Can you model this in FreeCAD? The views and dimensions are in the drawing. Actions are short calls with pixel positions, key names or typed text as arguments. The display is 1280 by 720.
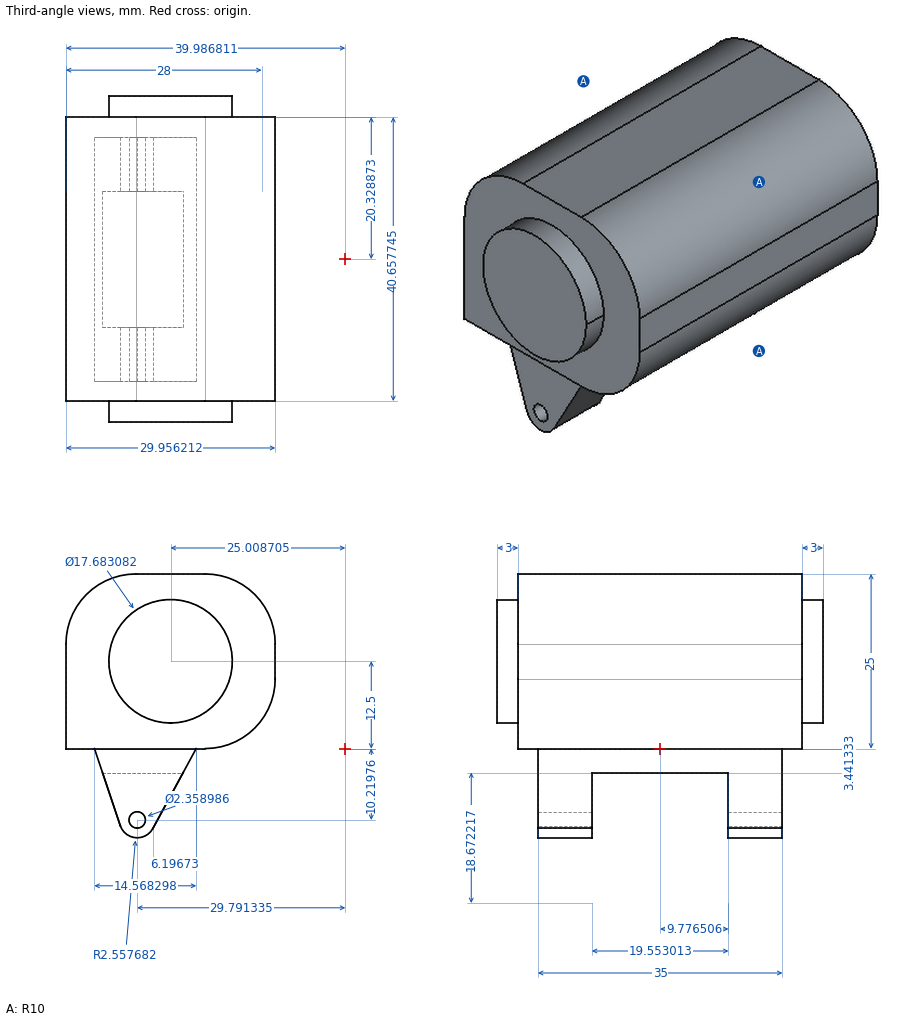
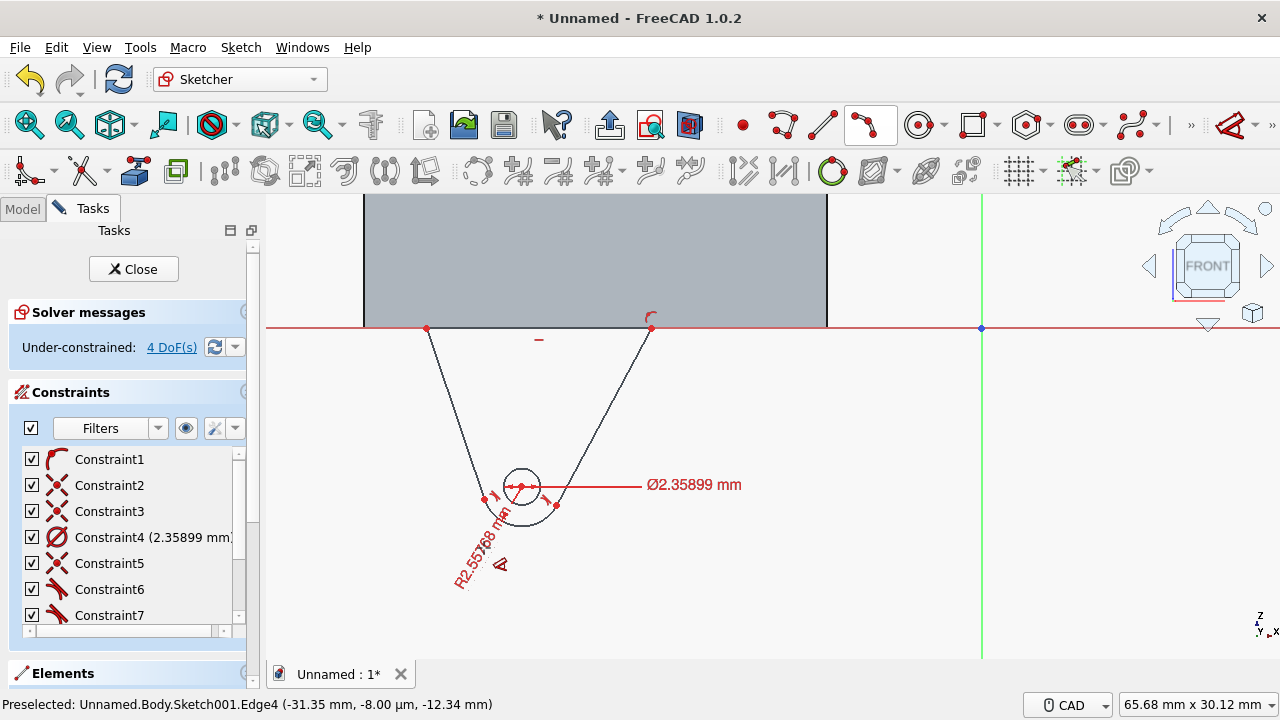
click(585, 452)
click(604, 294)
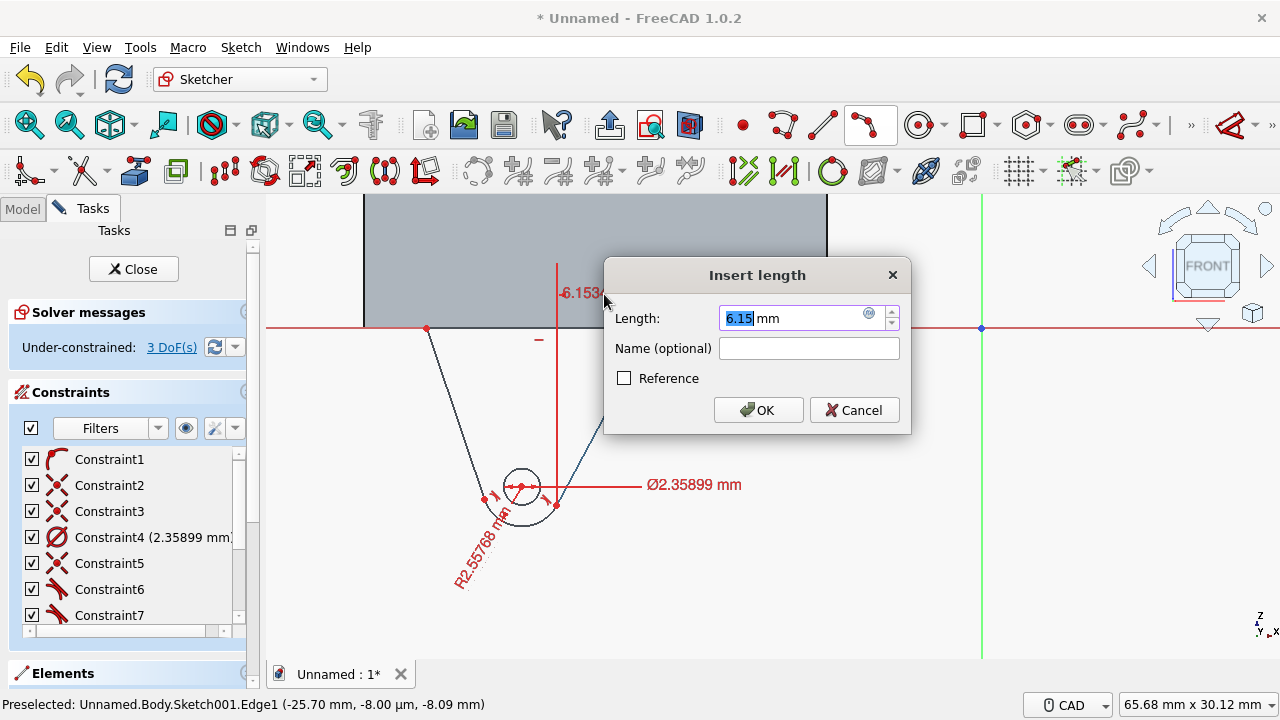
text(6.19673)
key(Return)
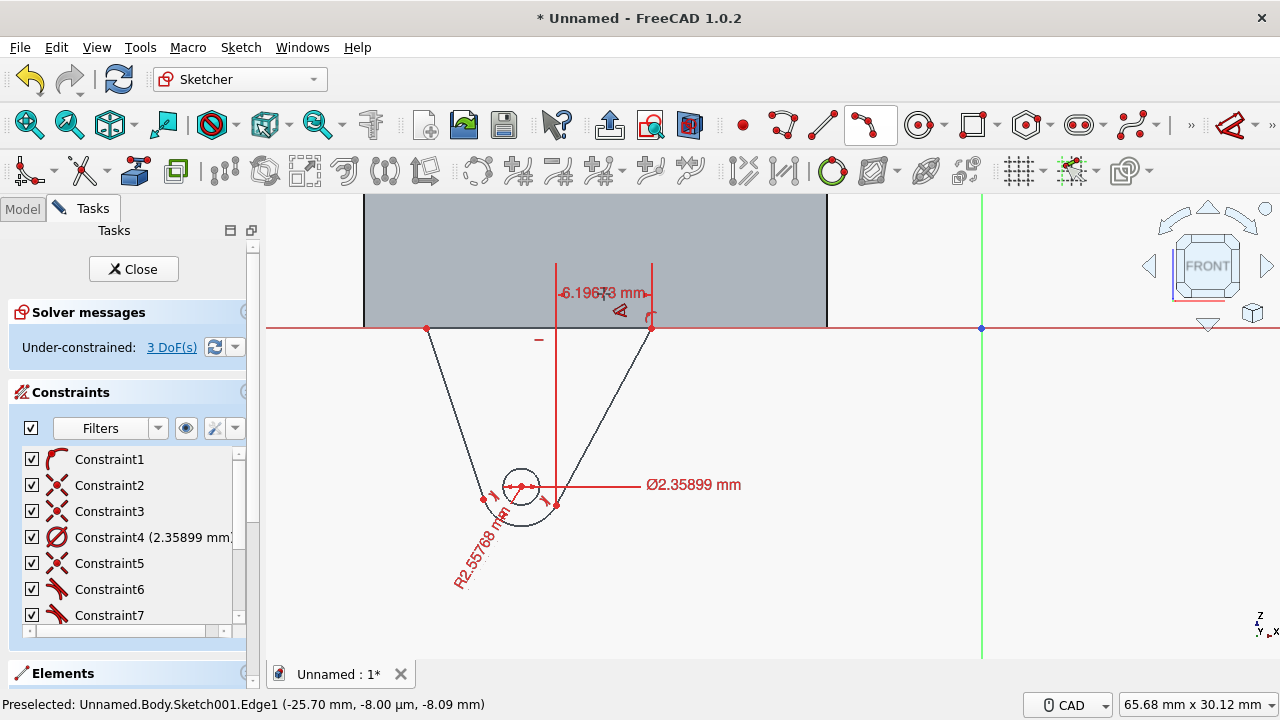
click(521, 487)
click(1016, 407)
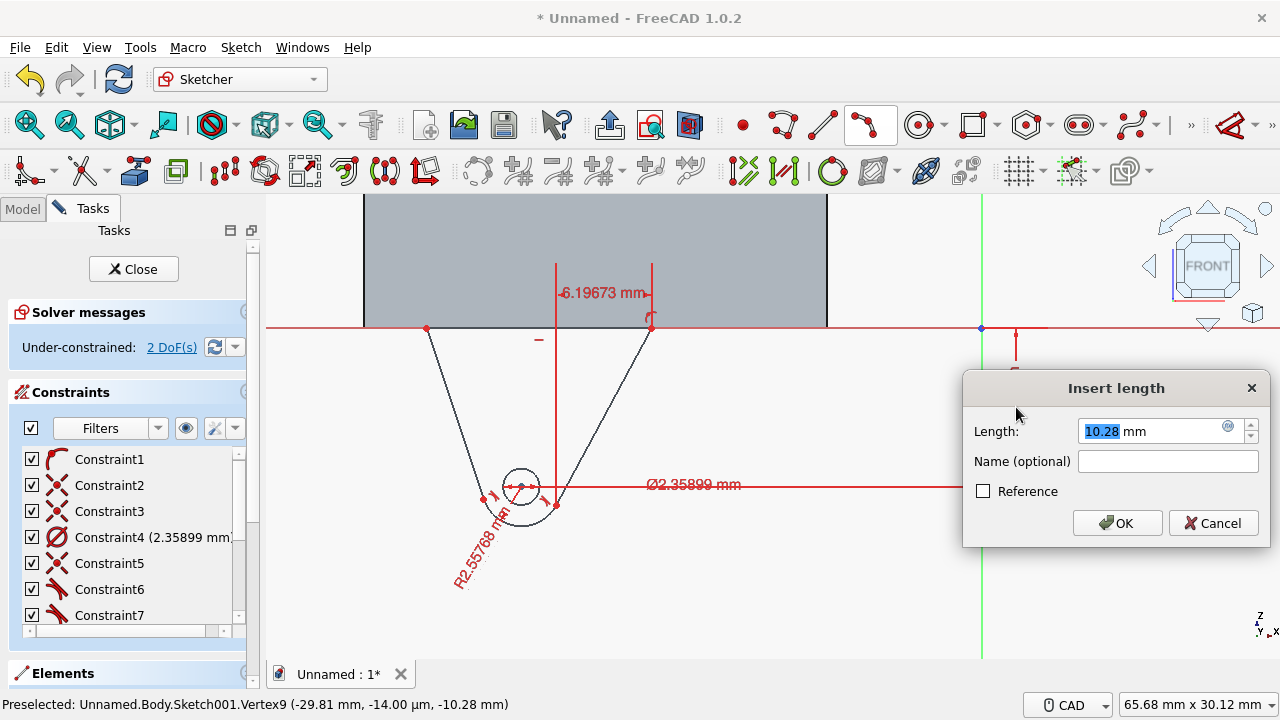
text(10.21976)
key(Return)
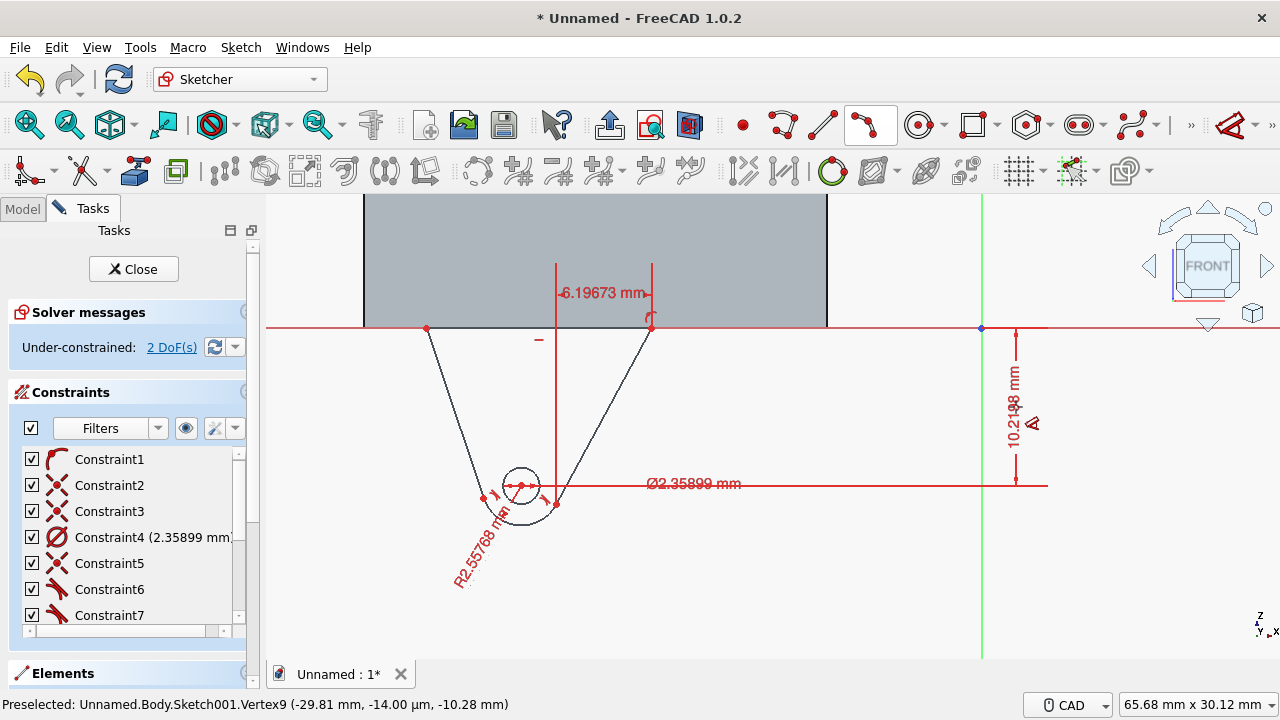
click(584, 328)
click(488, 294)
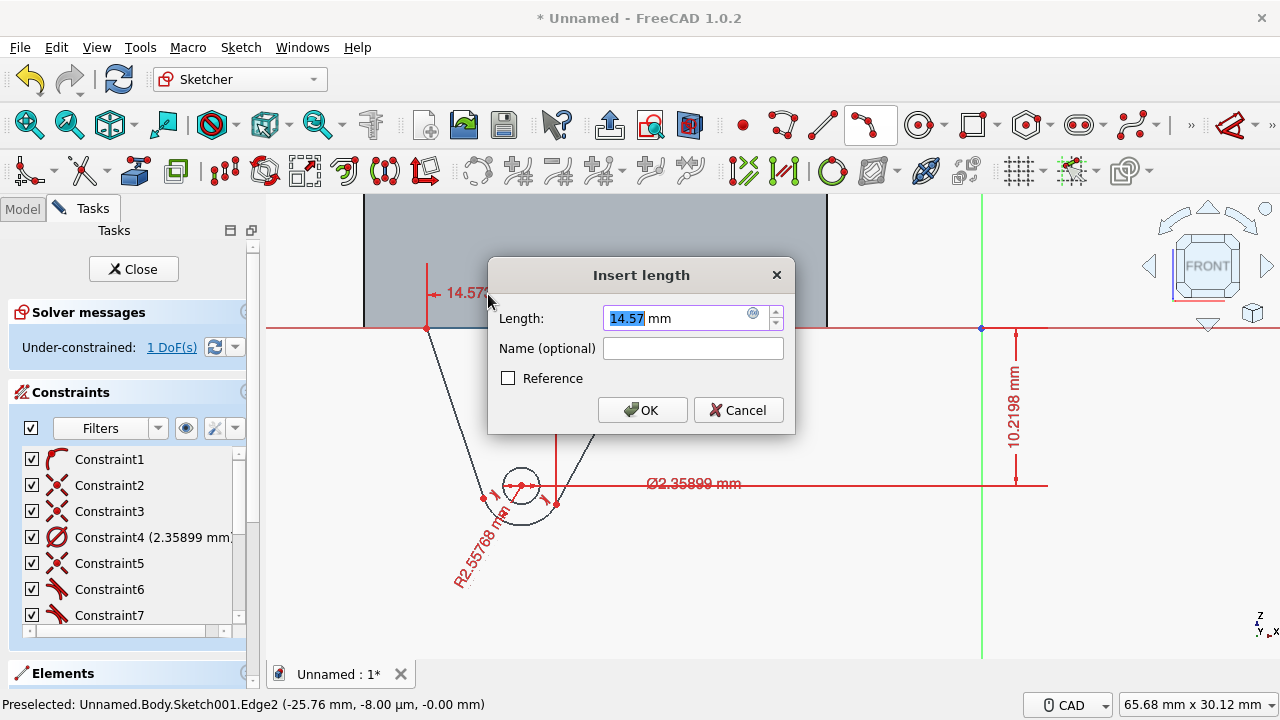
text(14.568298)
key(Return)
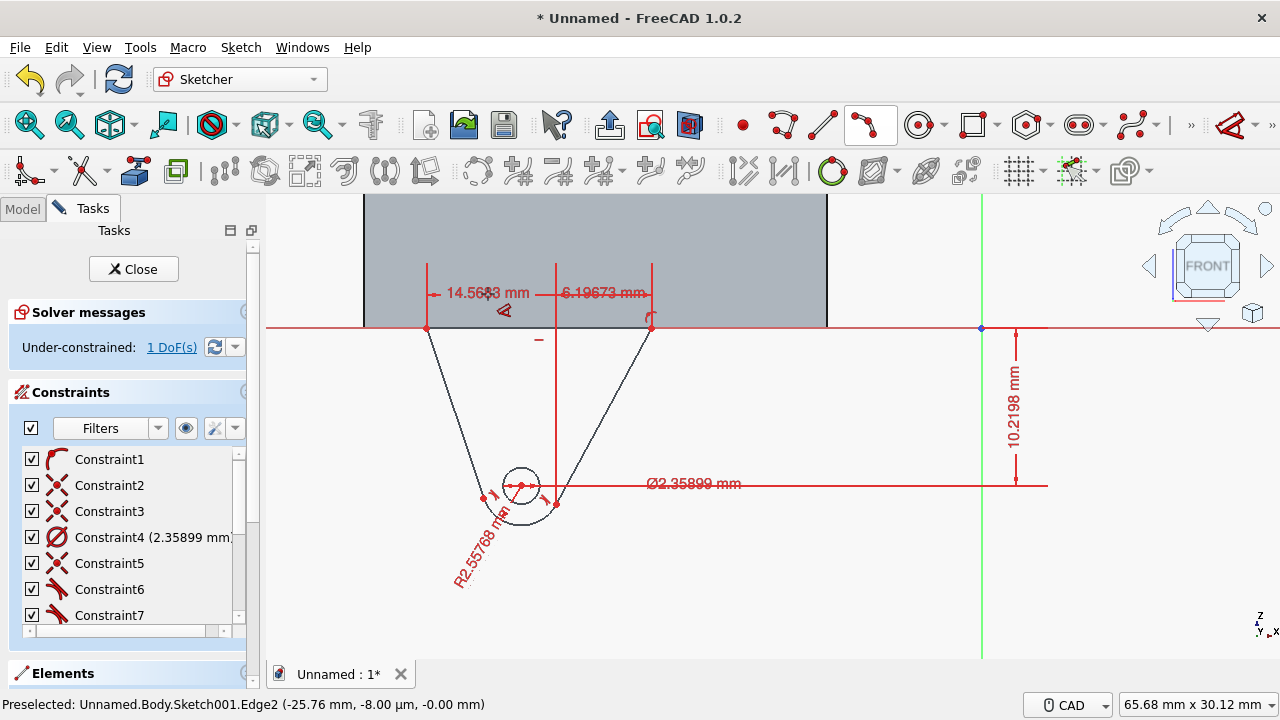
click(521, 486)
click(752, 294)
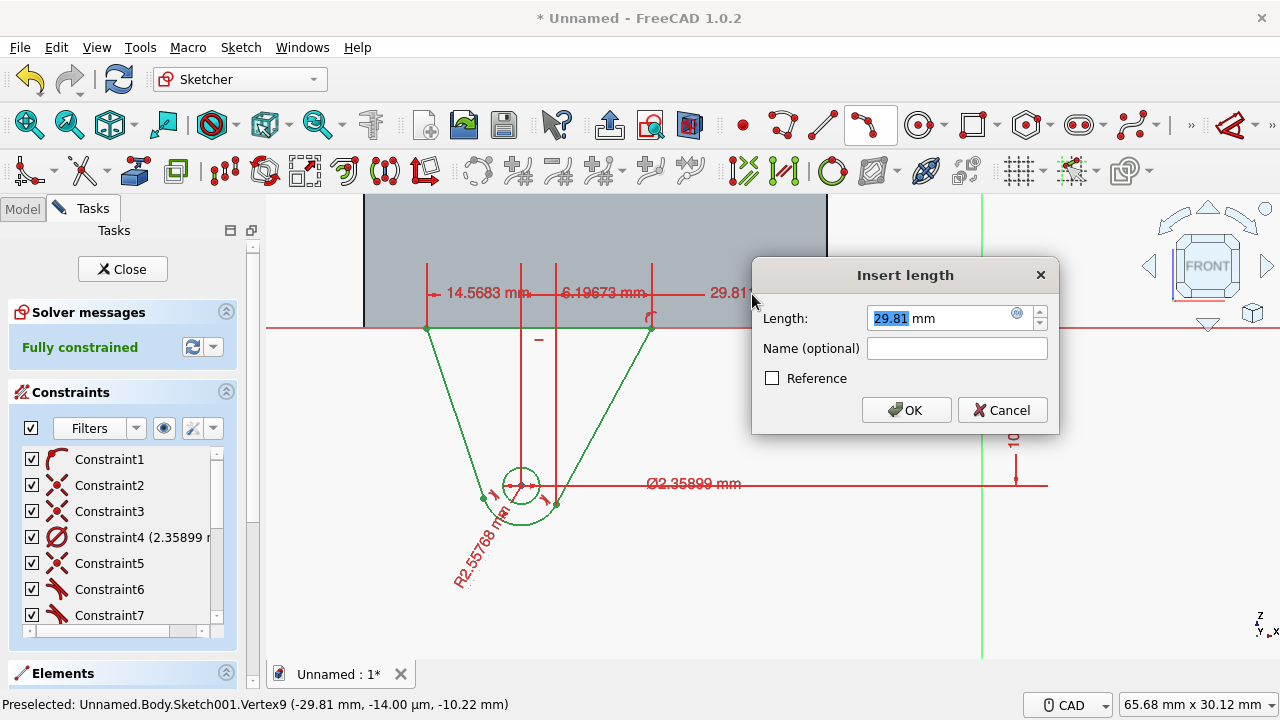
text(29.791335)
key(Return)
key(Escape)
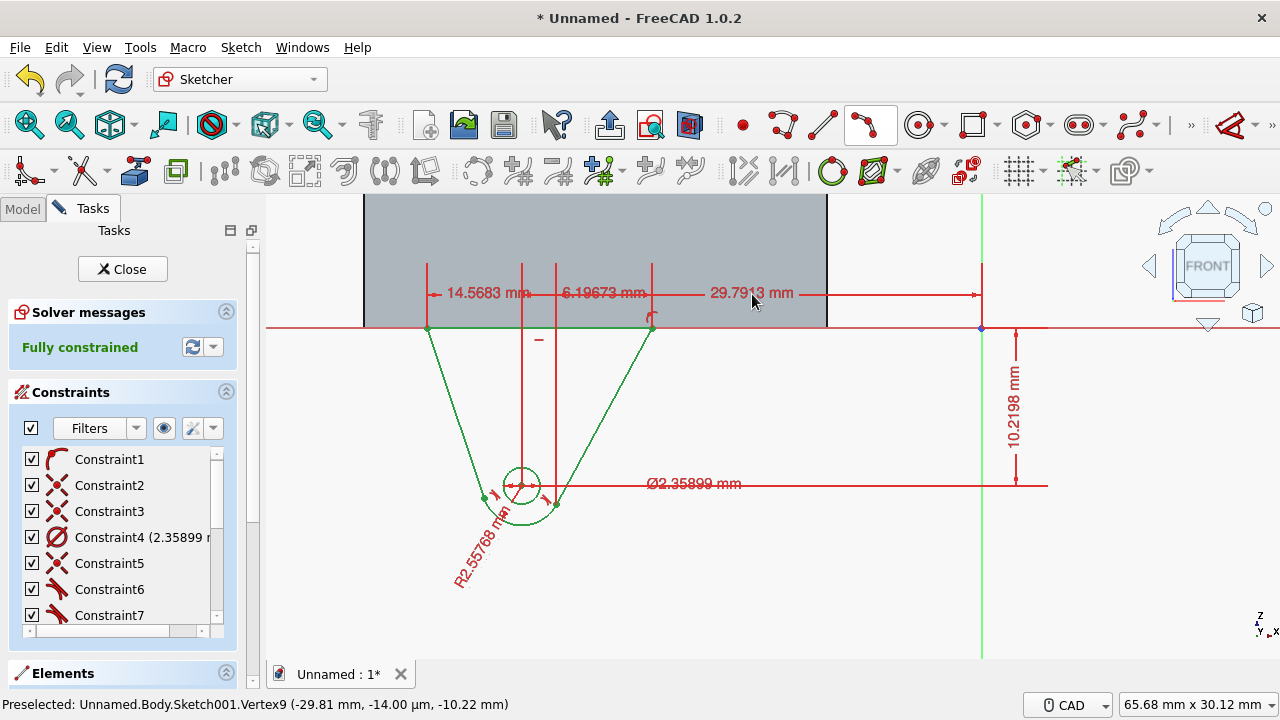
click(123, 269)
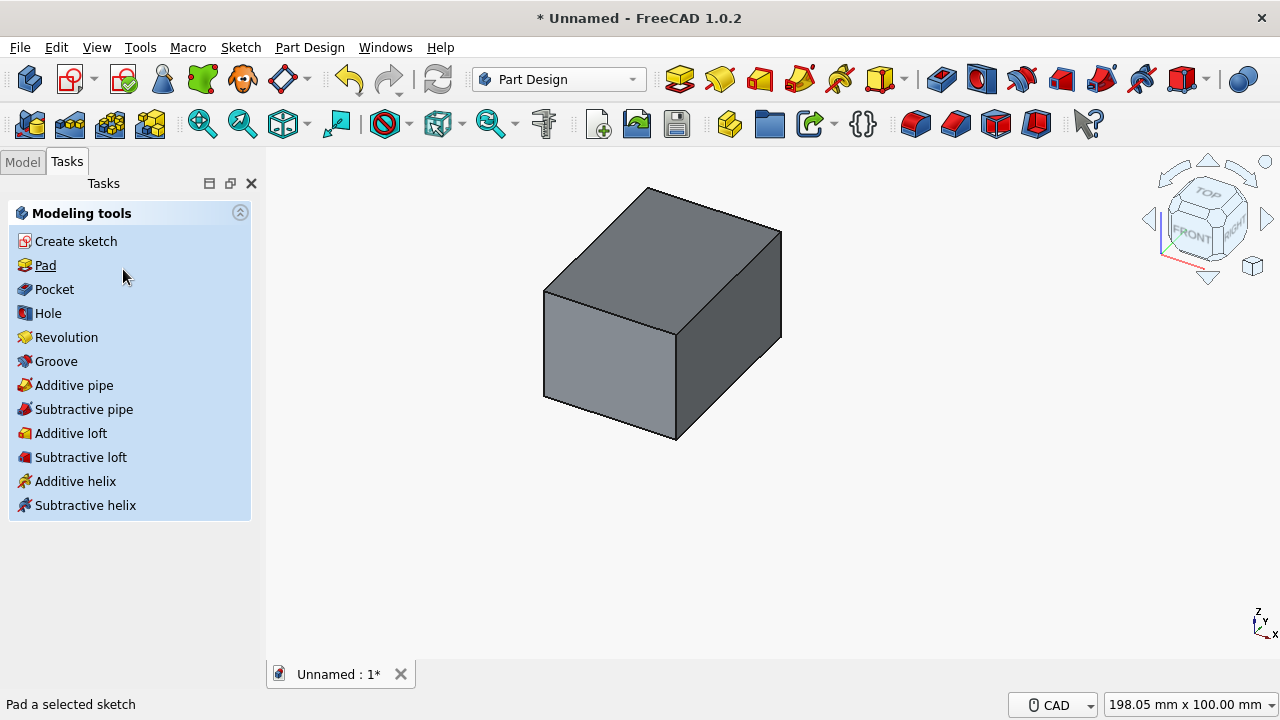
click(680, 80)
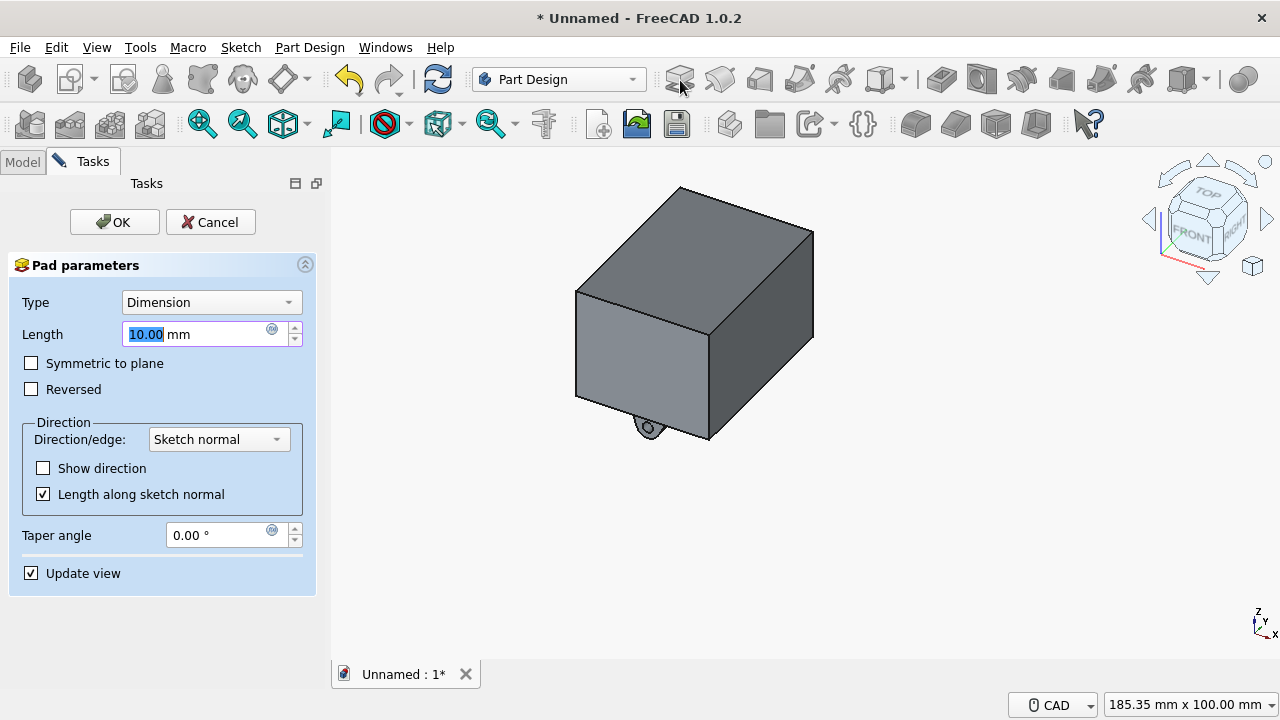
text(35)
key(Tab)